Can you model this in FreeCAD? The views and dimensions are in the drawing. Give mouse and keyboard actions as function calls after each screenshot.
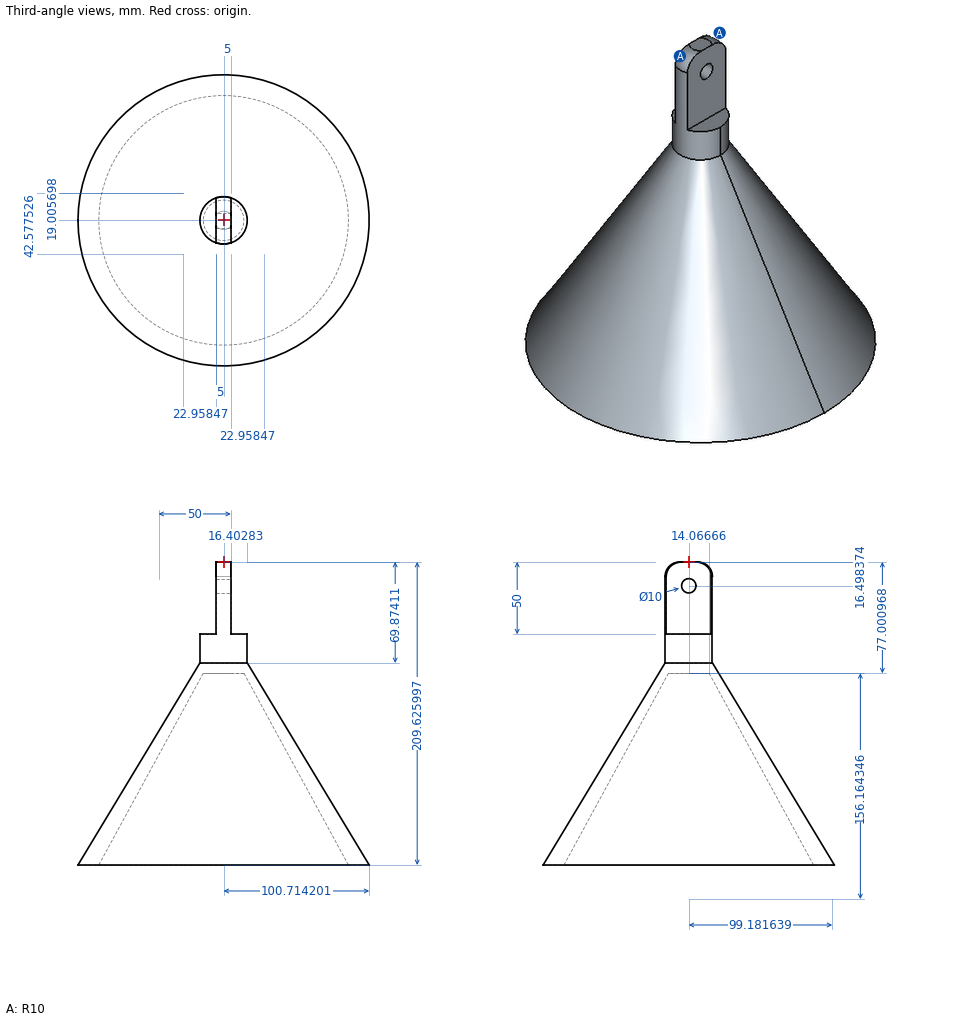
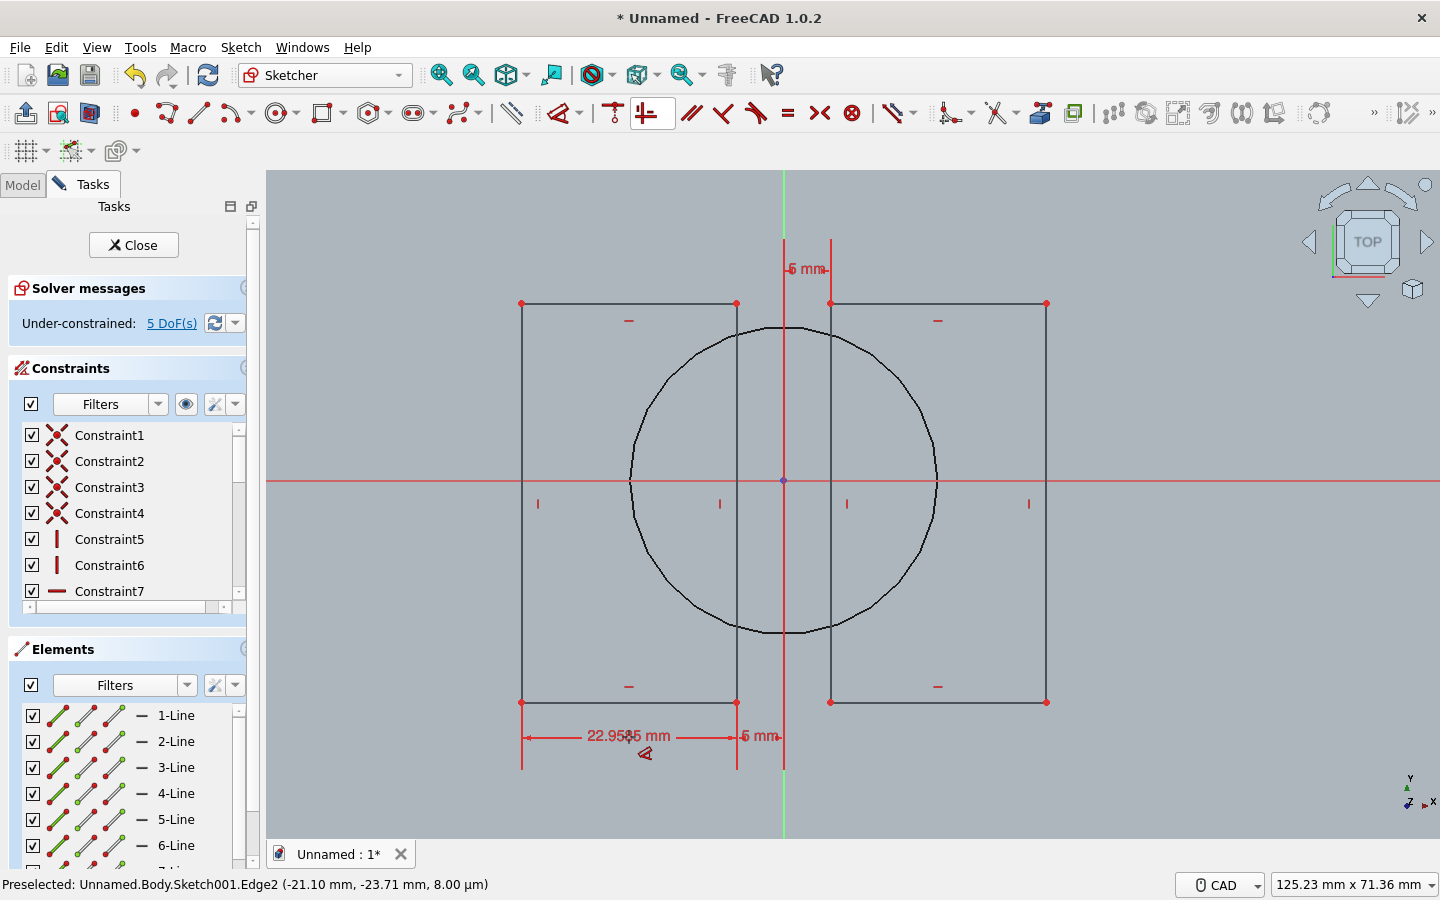
click(895, 703)
click(938, 737)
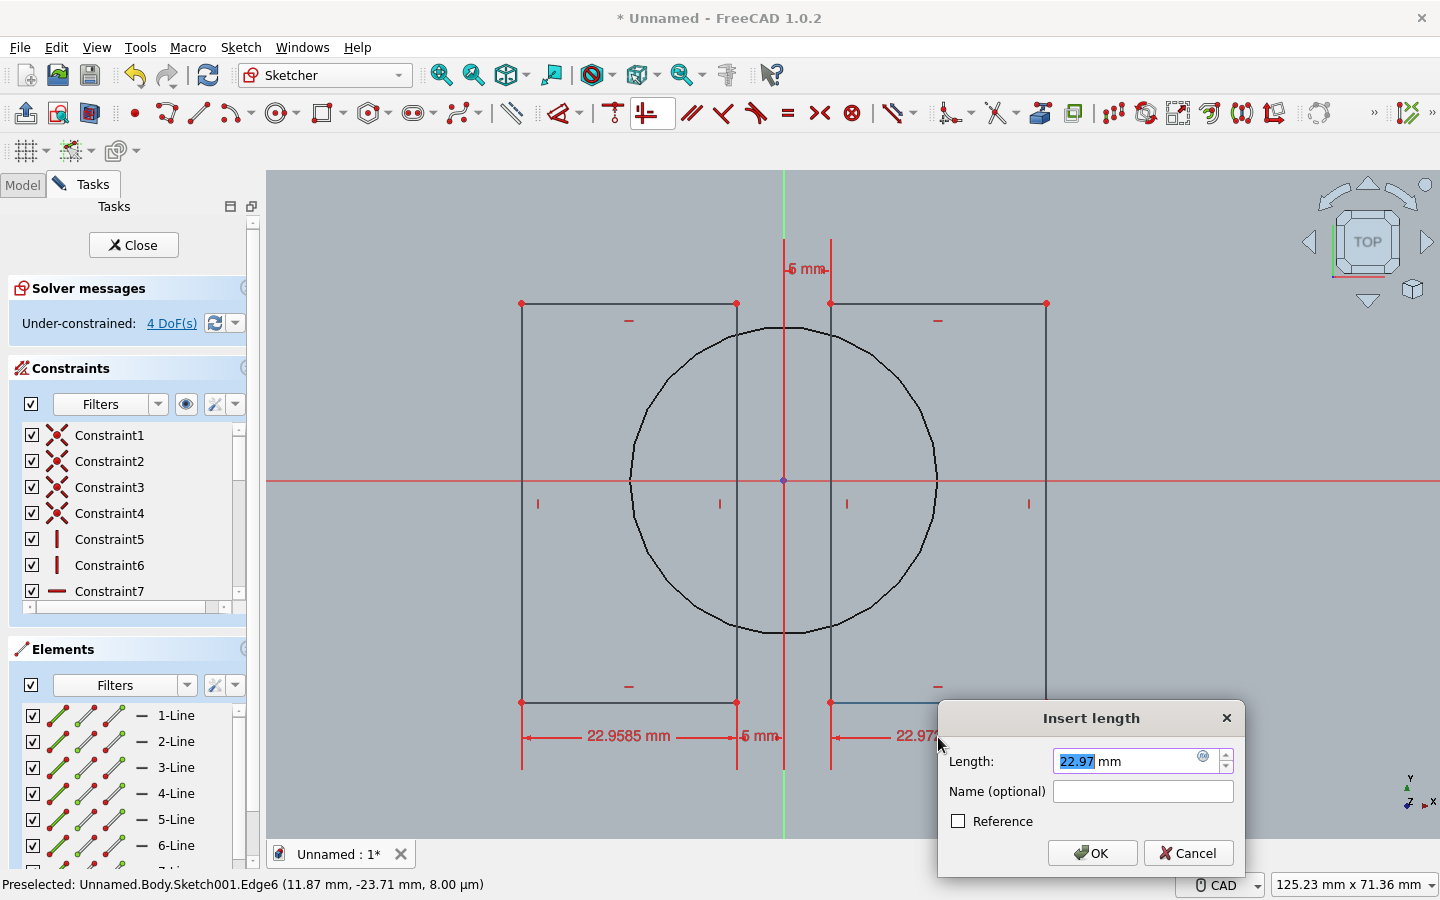
text(22.95847)
key(Return)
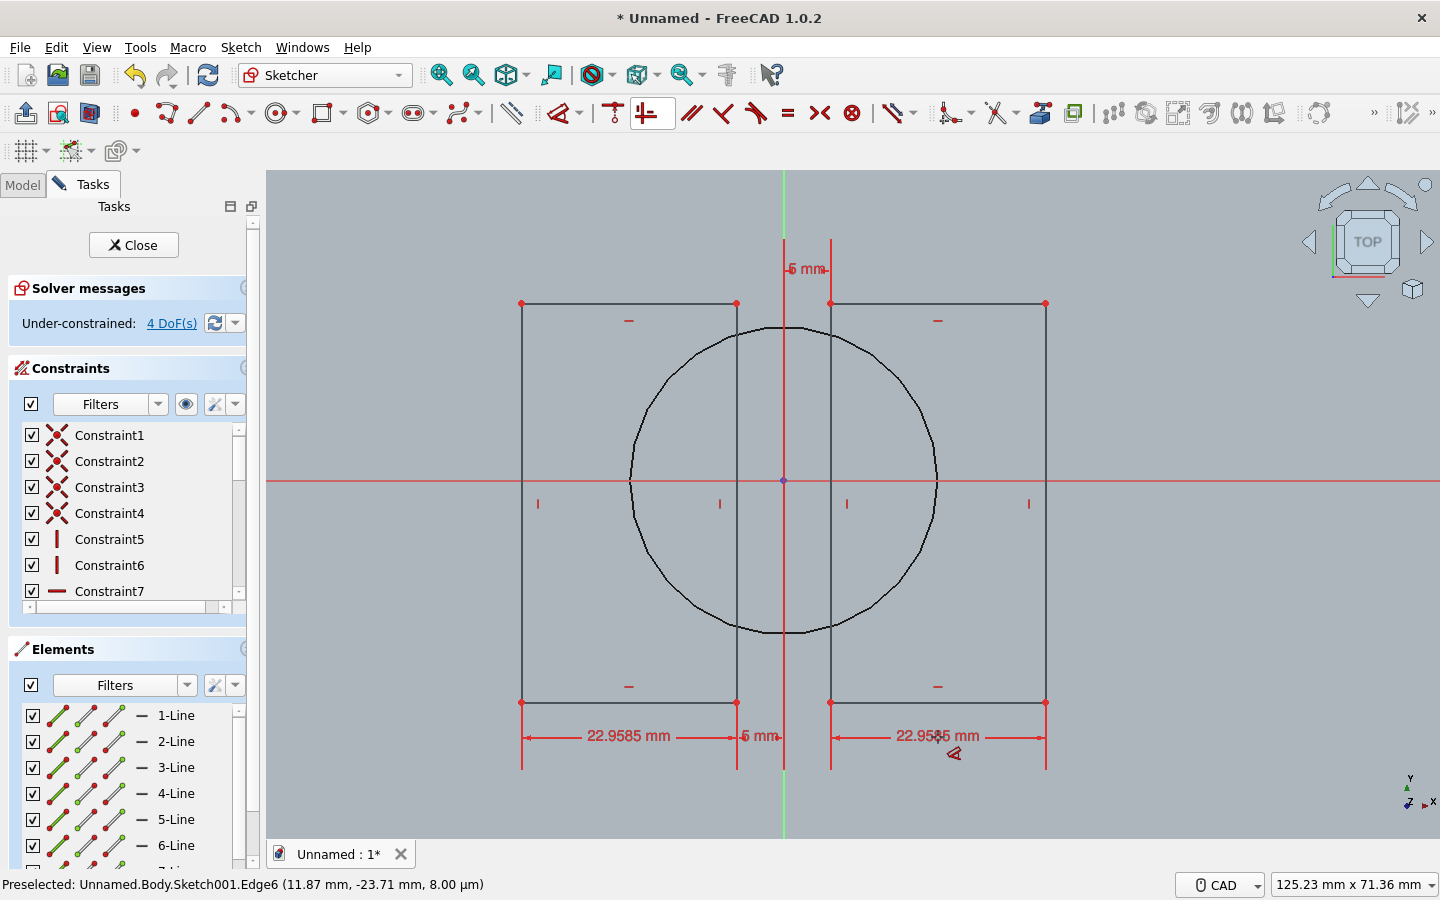
click(522, 424)
click(488, 504)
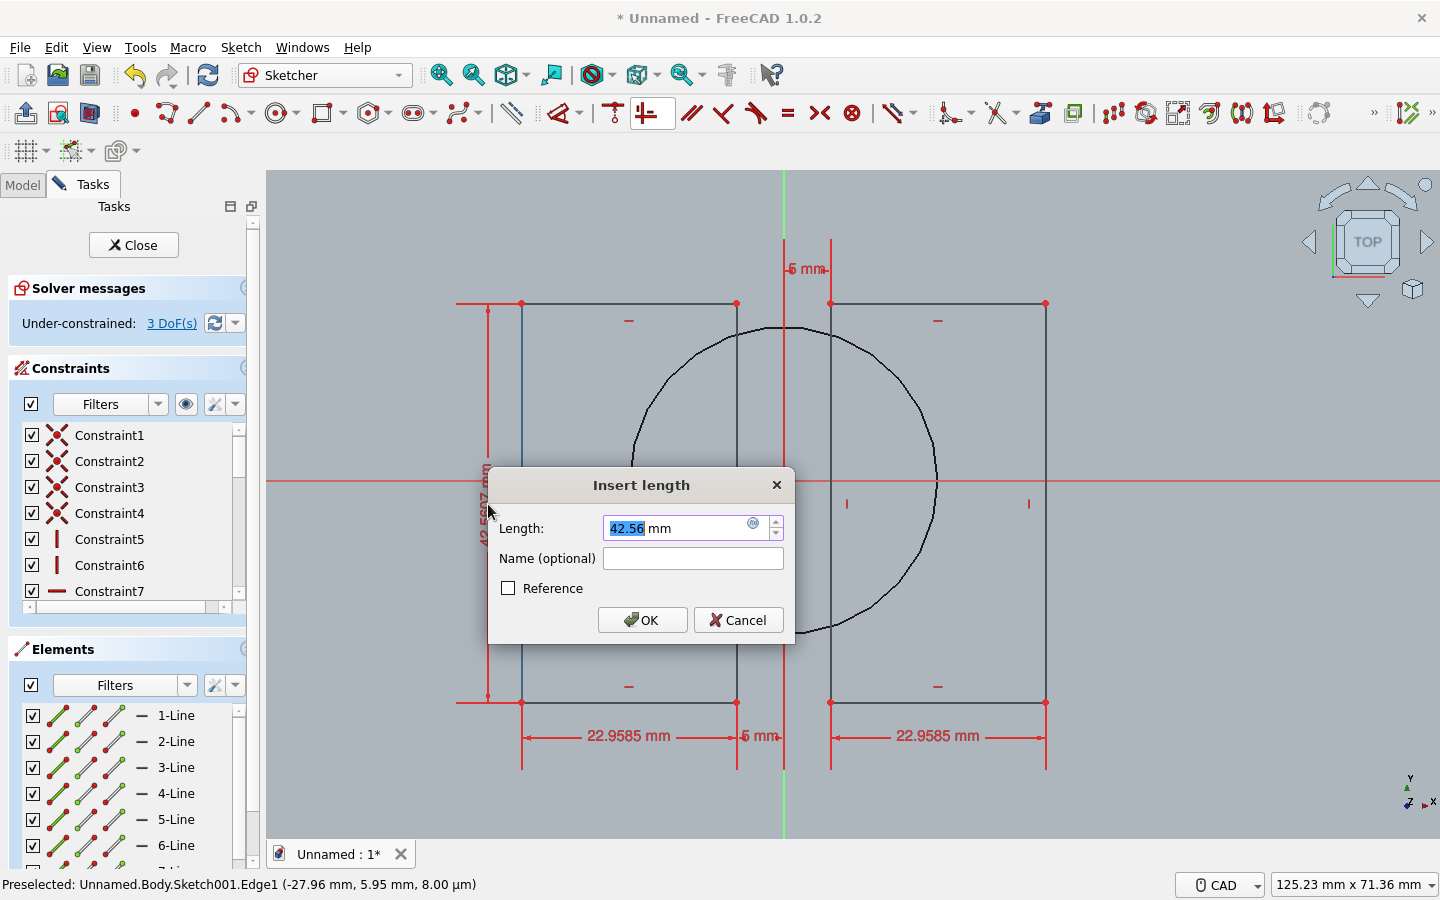
text(42.577526)
key(Return)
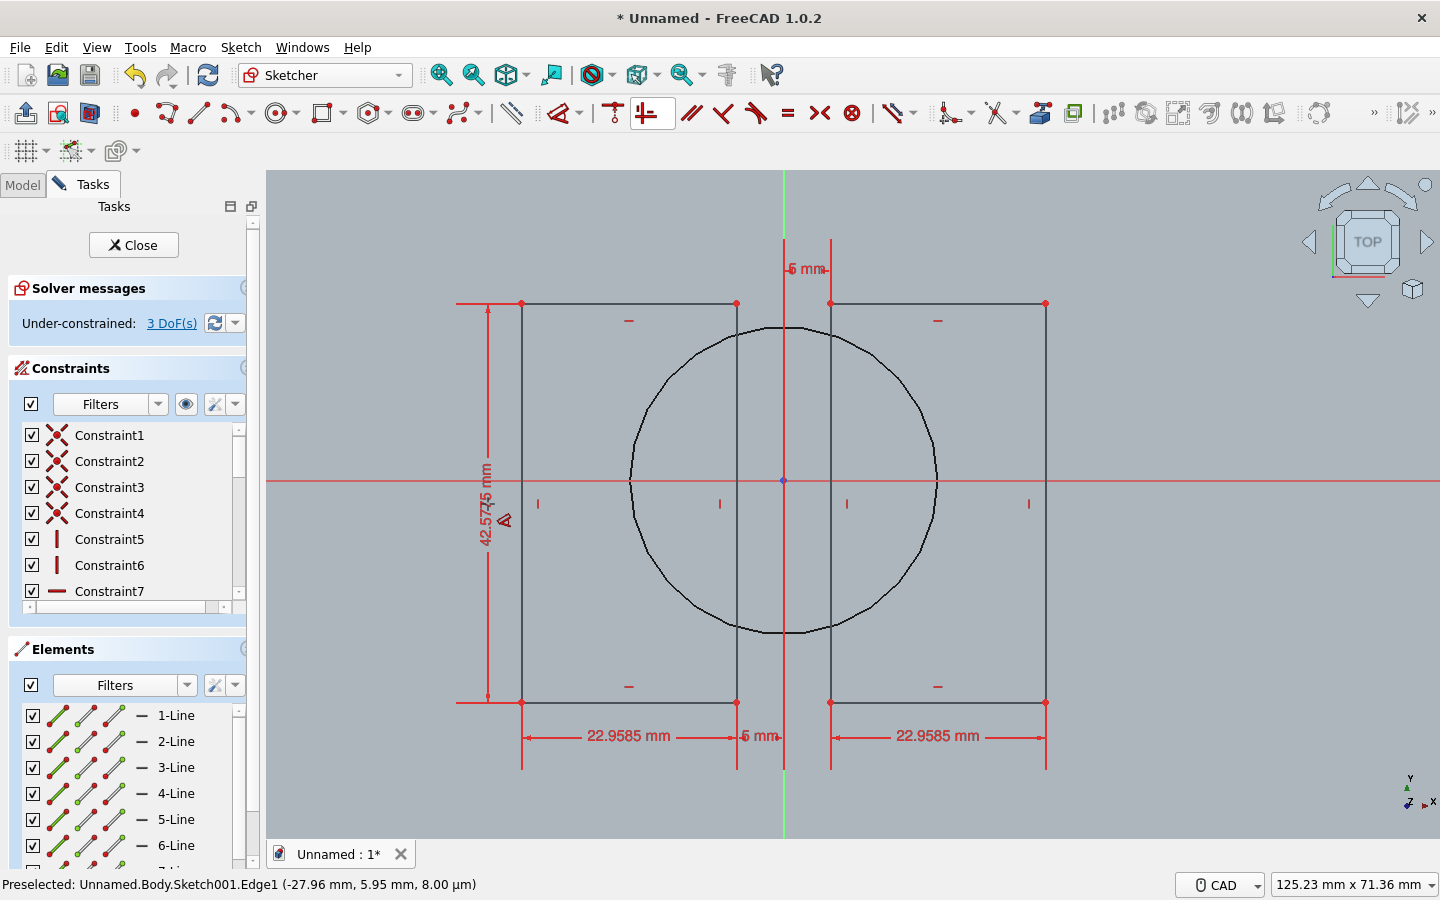
click(831, 424)
click(865, 504)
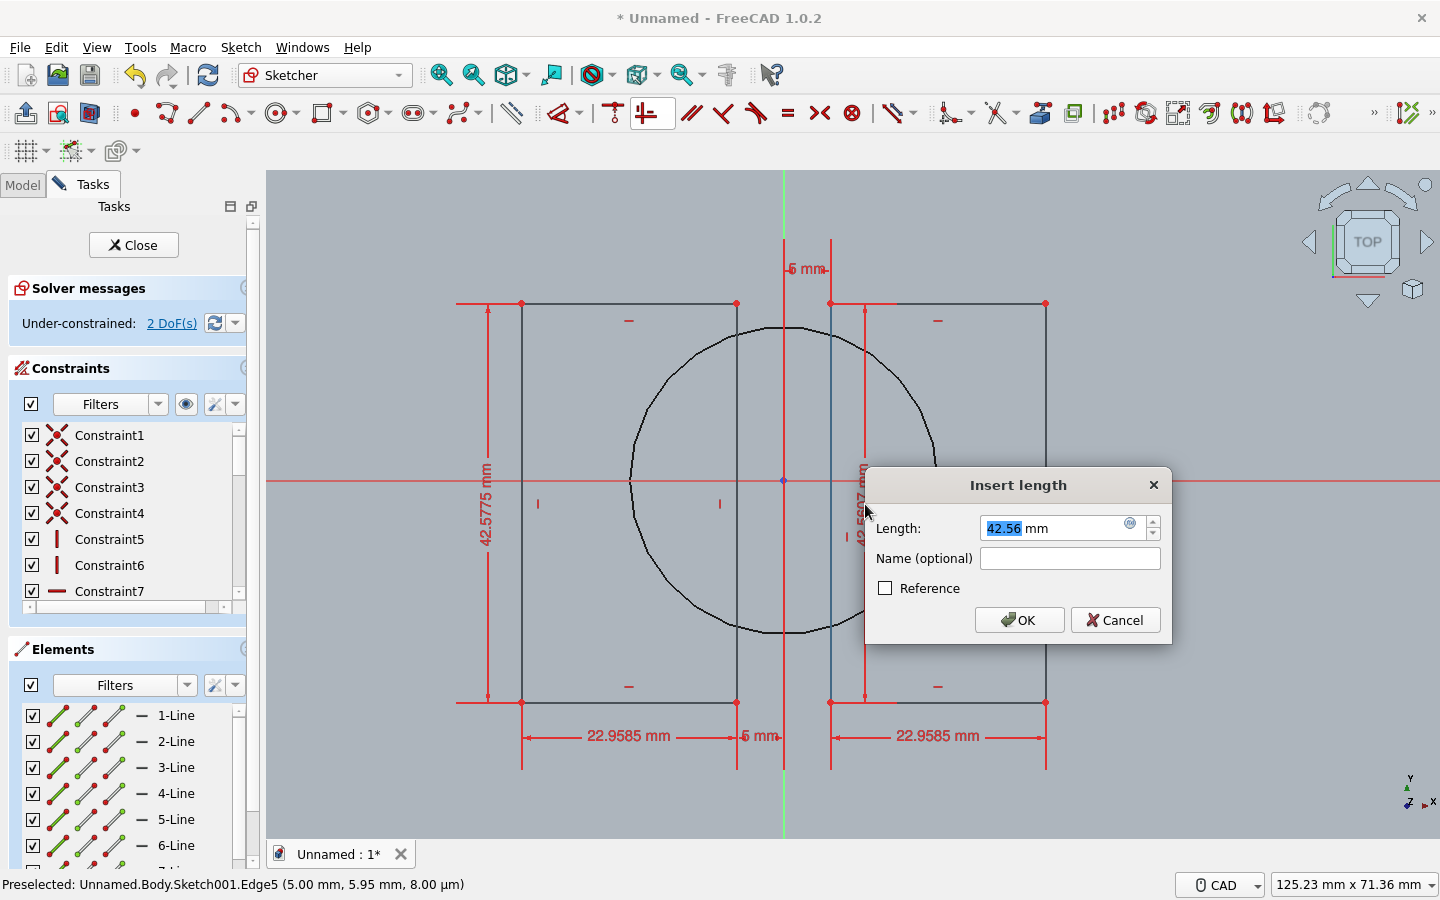
text(42.577526)
key(Return)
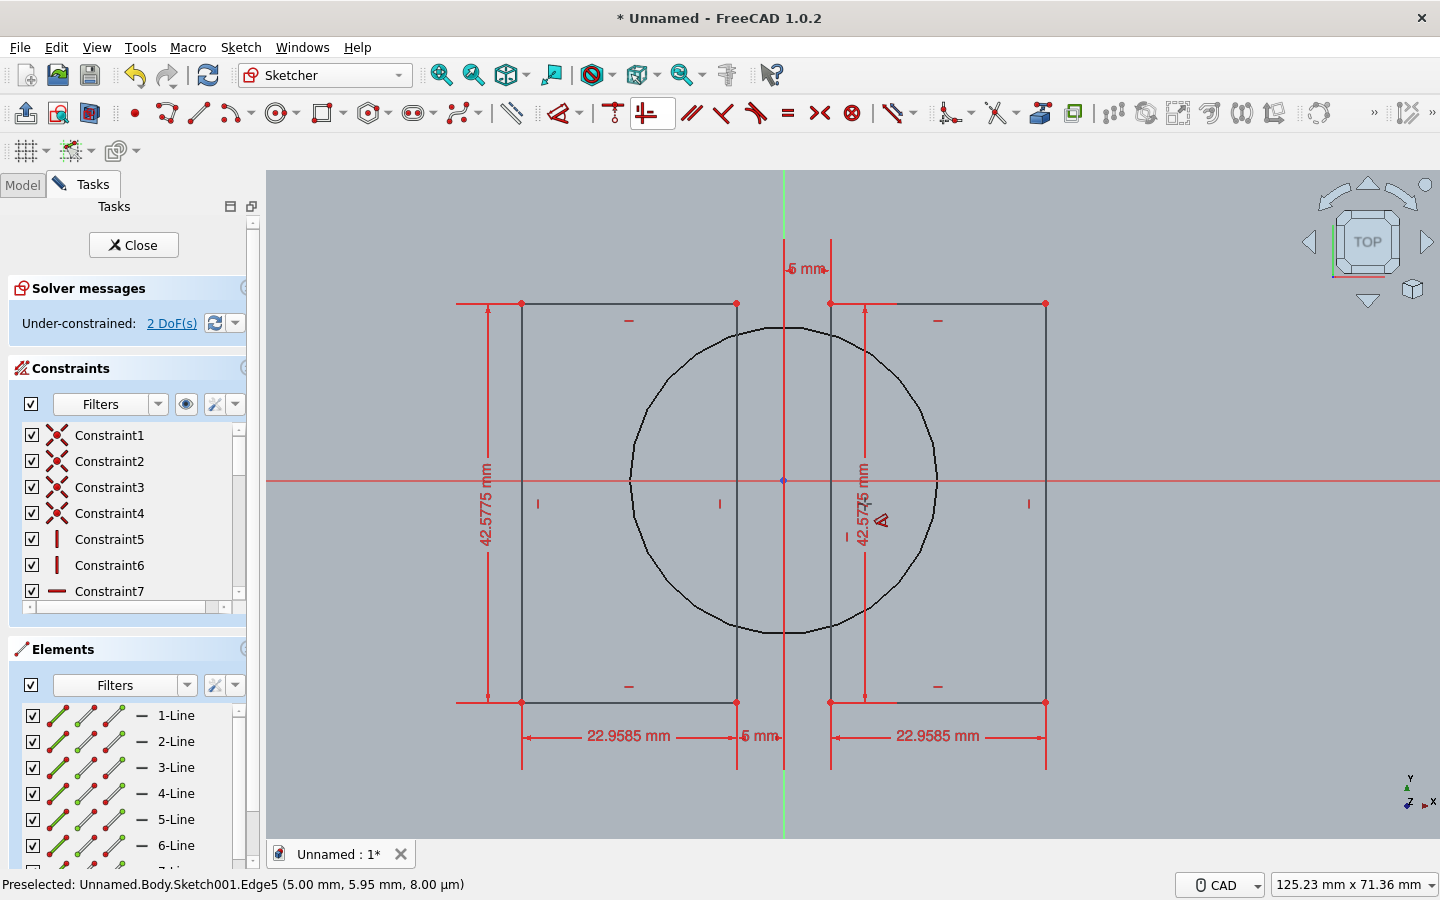
click(522, 304)
click(488, 392)